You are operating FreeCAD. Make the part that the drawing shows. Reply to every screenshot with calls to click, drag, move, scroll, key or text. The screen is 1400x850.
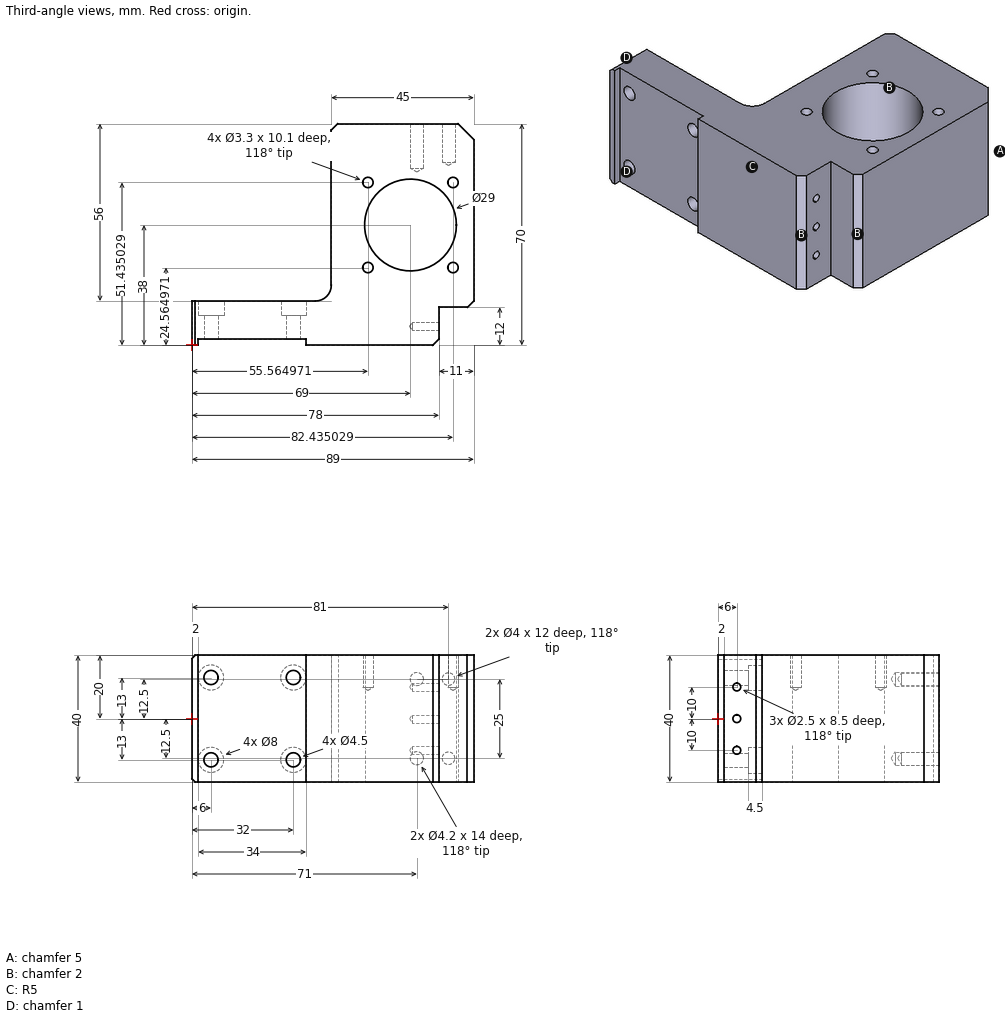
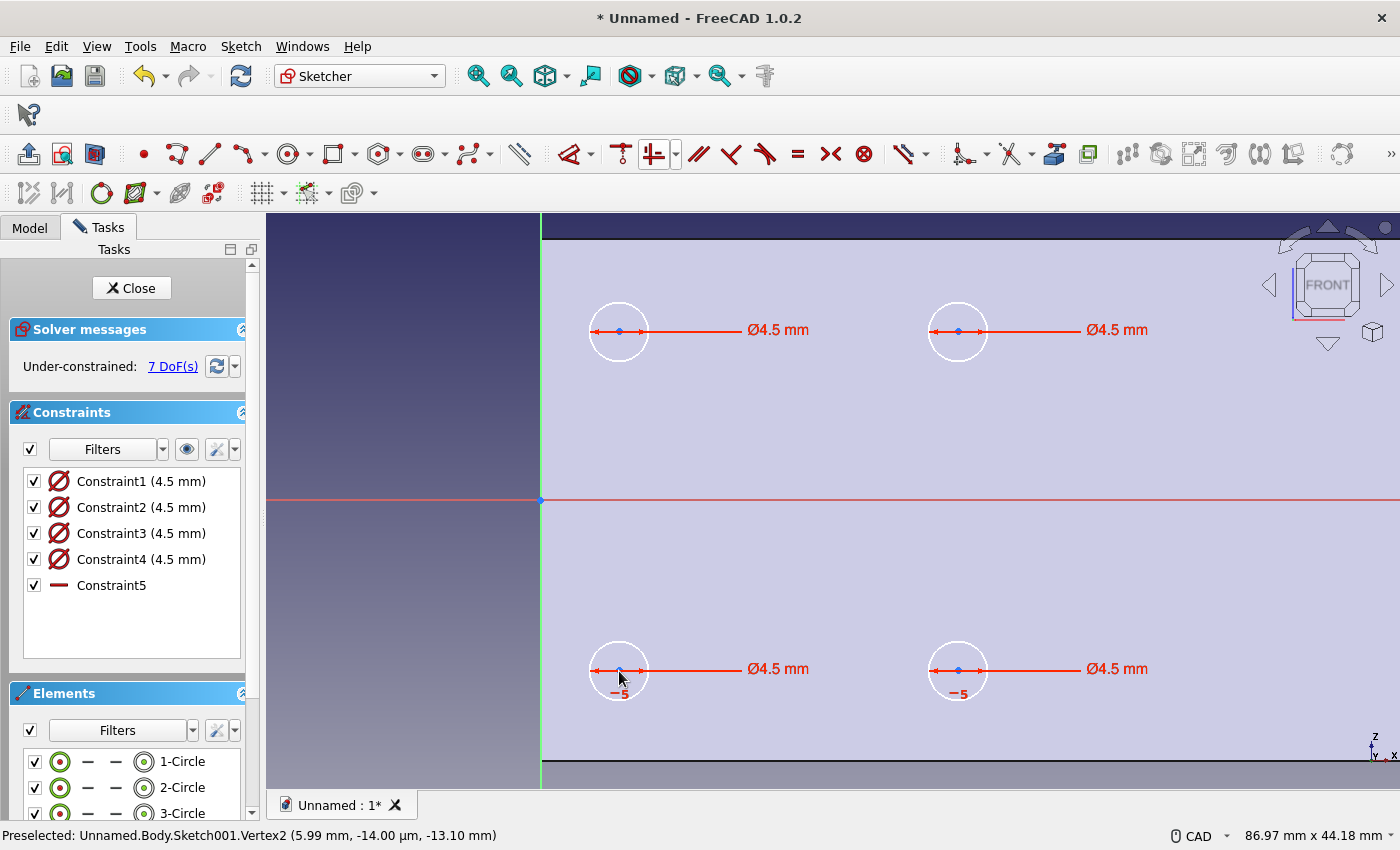
click(619, 671)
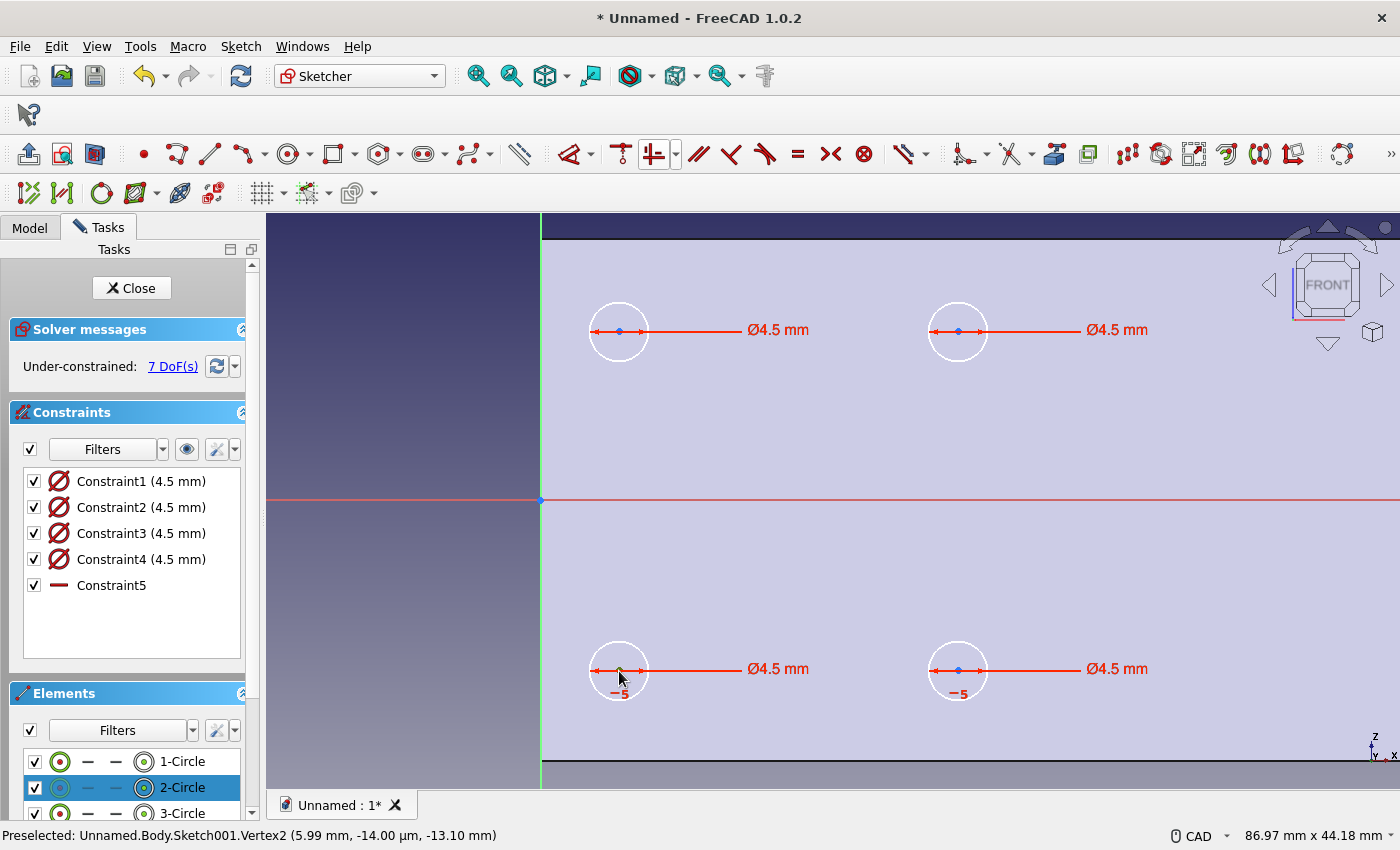
click(619, 332)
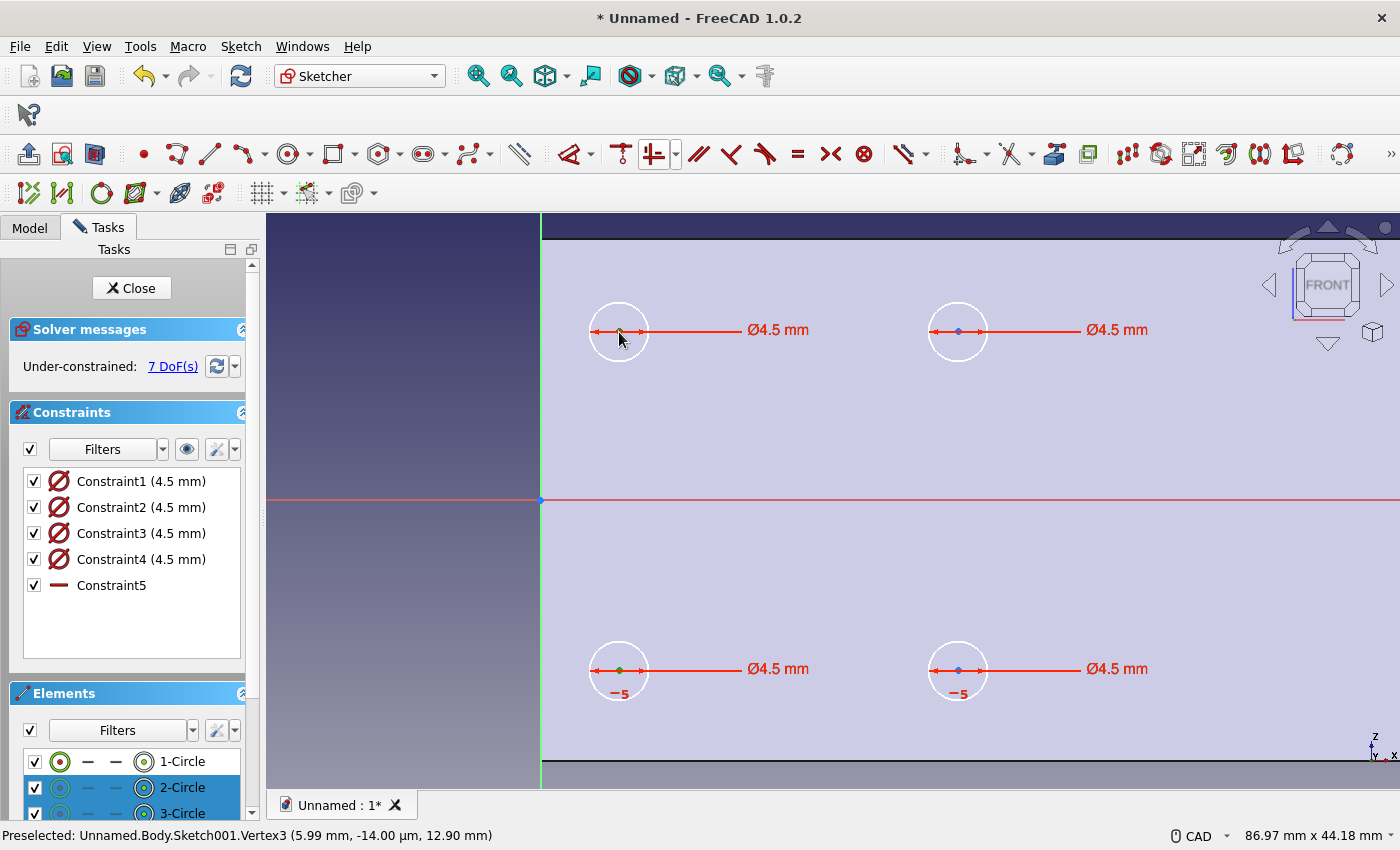
click(676, 154)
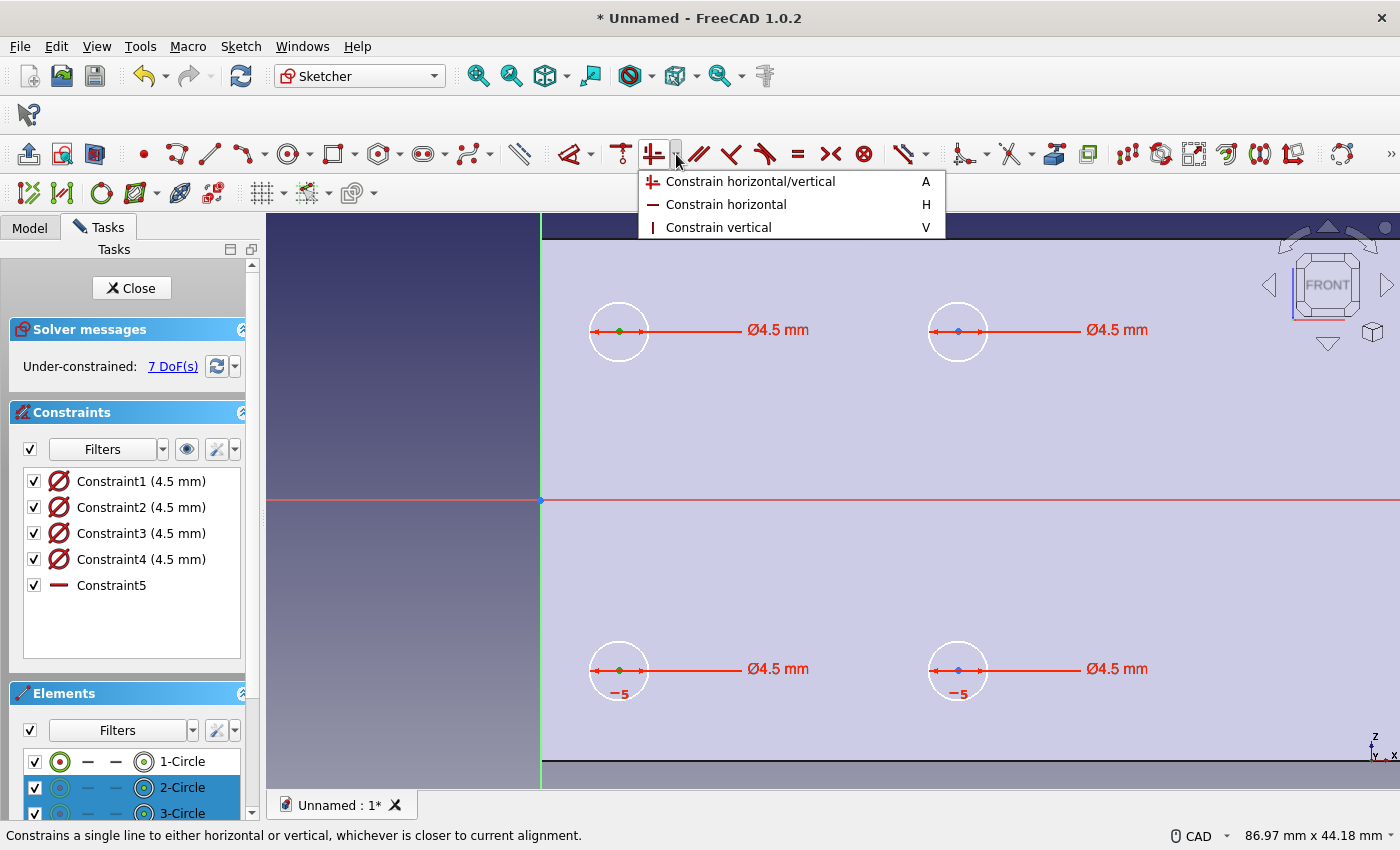
click(792, 228)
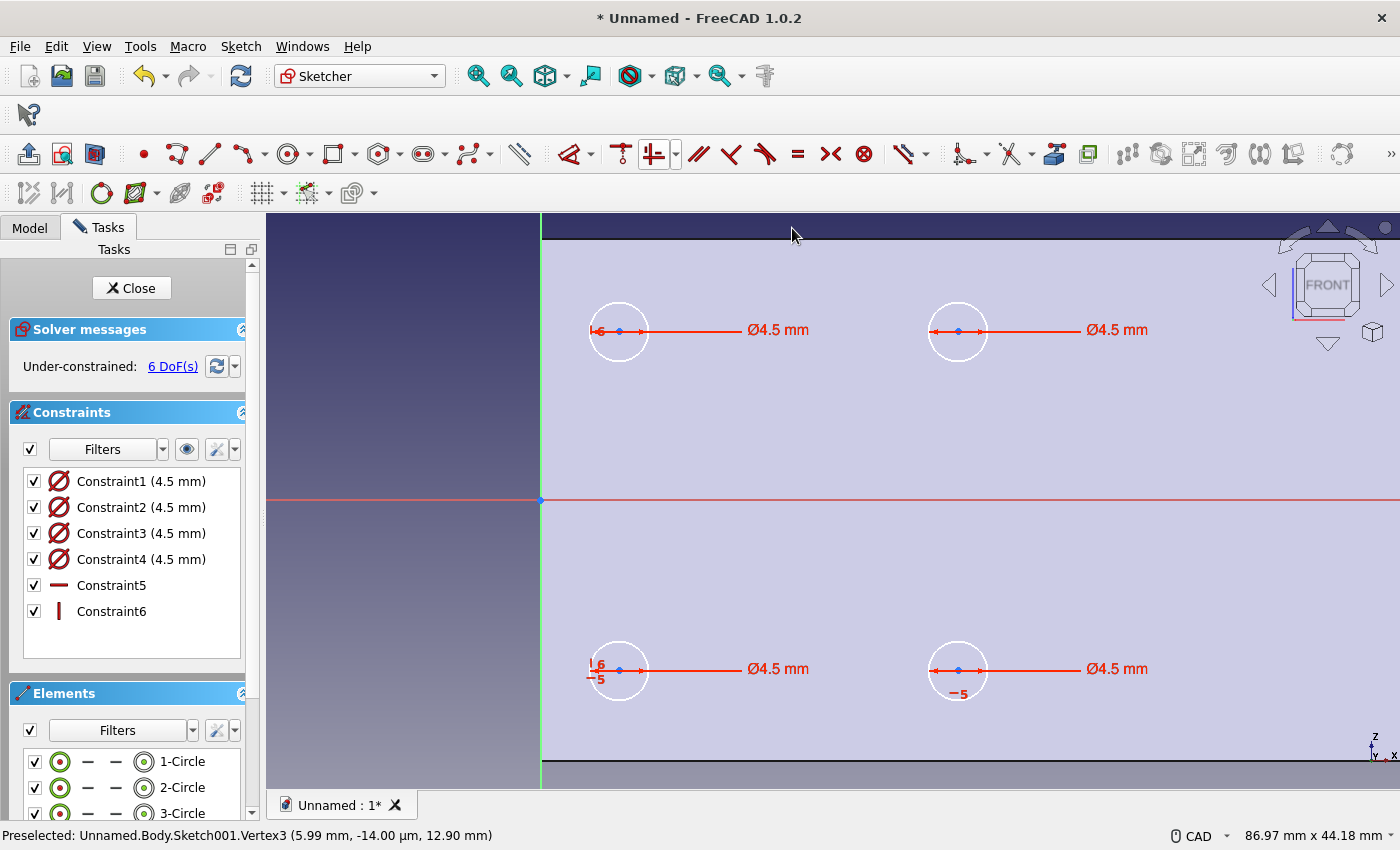
click(958, 671)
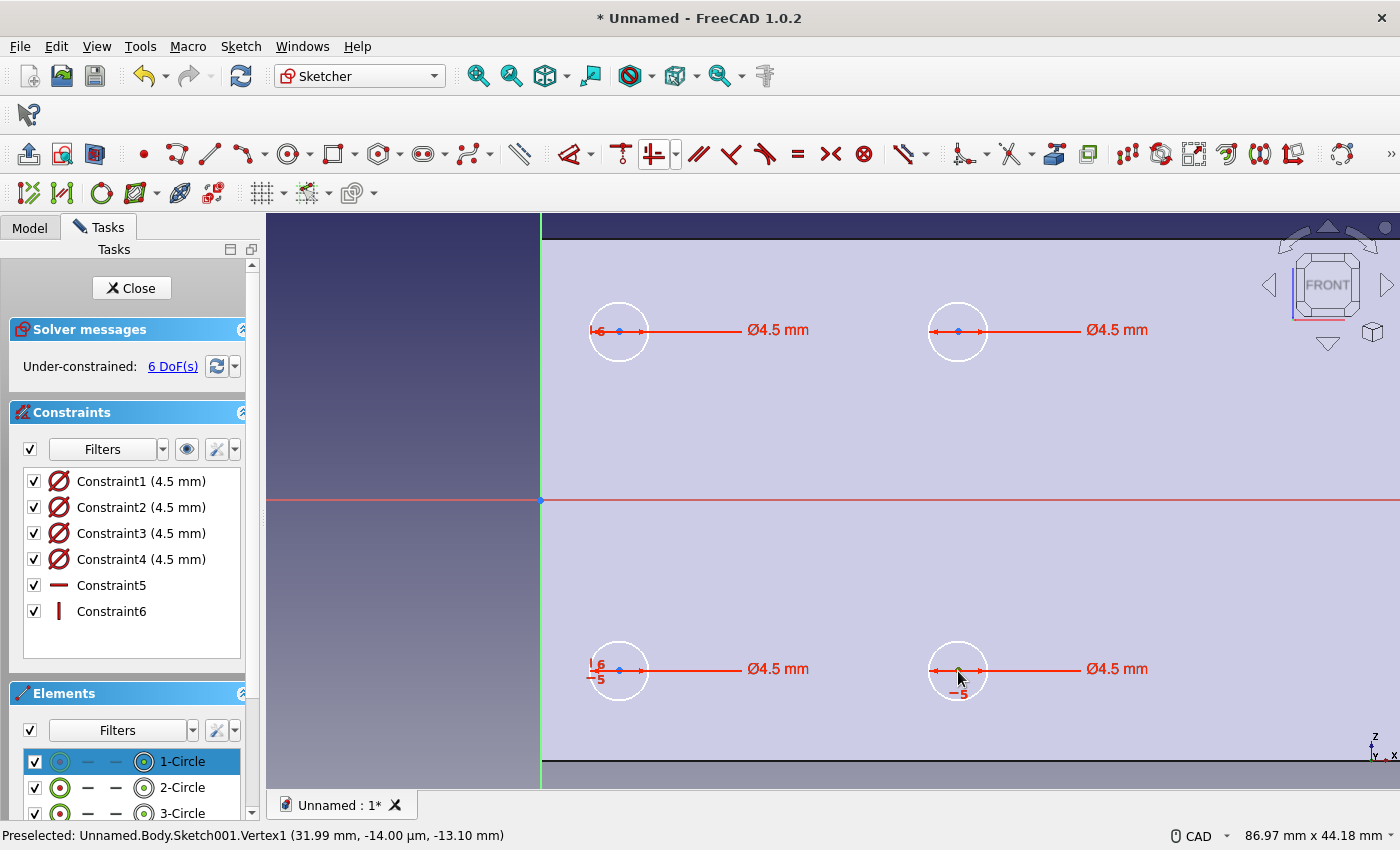
click(958, 332)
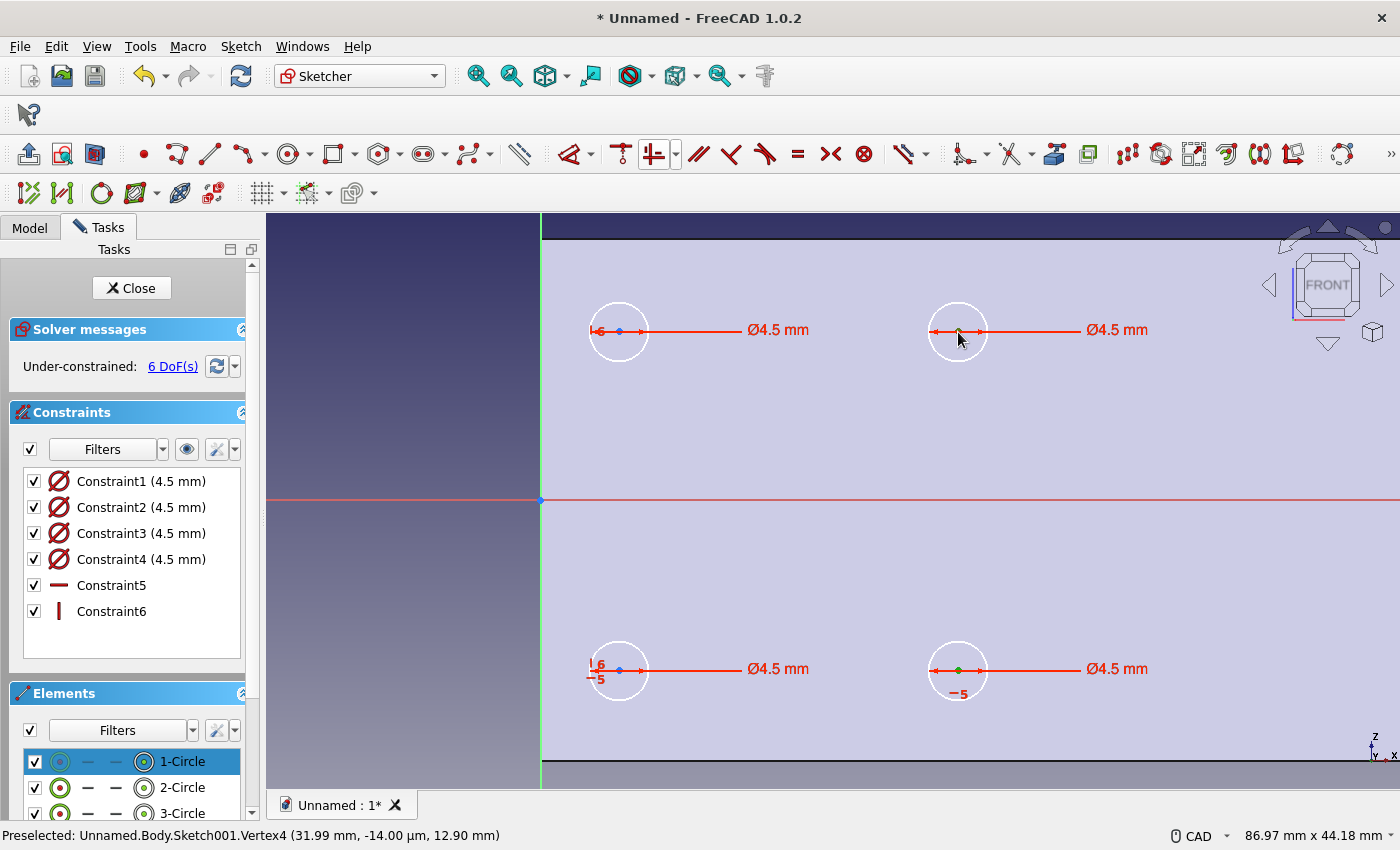
key(v)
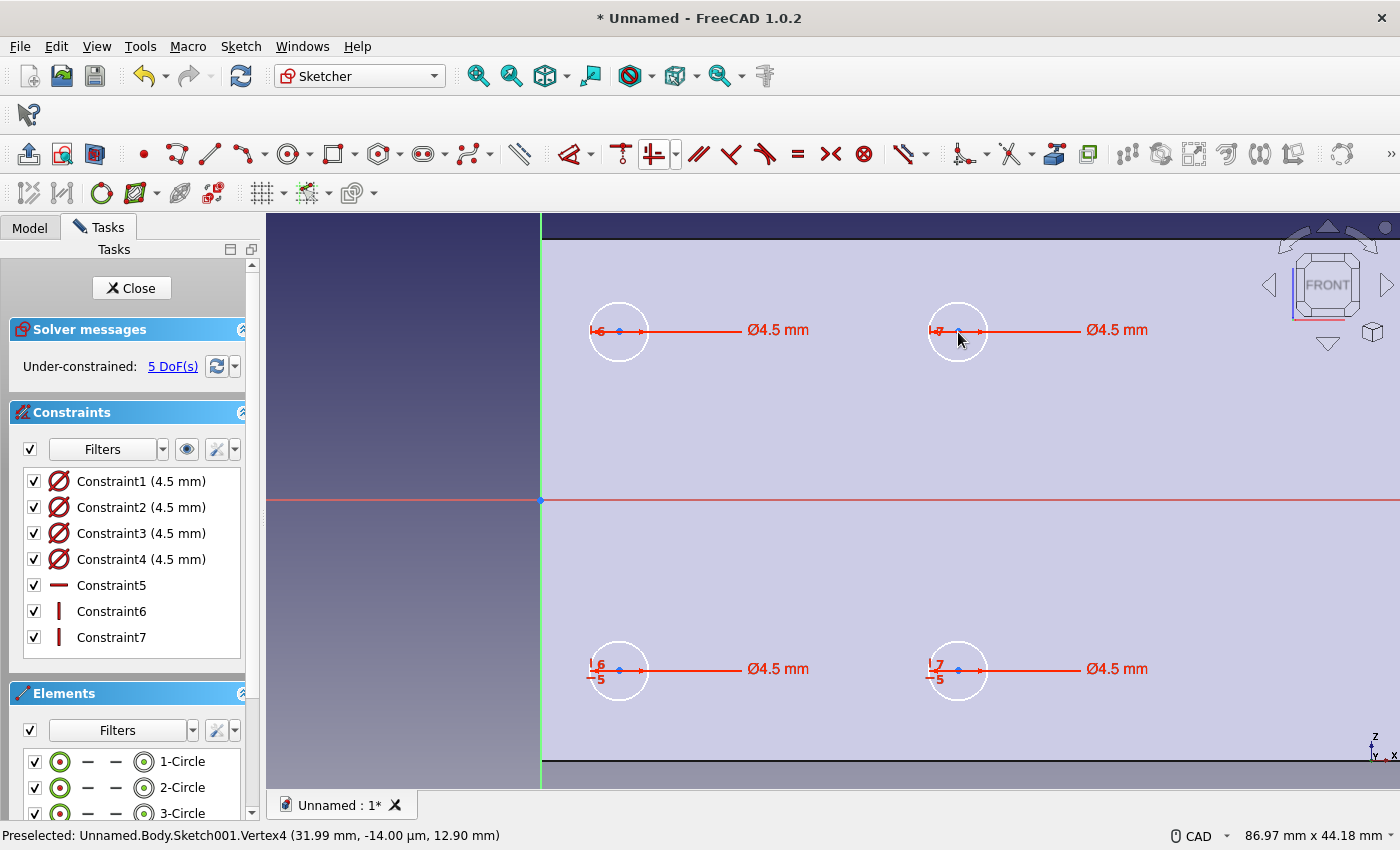
click(619, 332)